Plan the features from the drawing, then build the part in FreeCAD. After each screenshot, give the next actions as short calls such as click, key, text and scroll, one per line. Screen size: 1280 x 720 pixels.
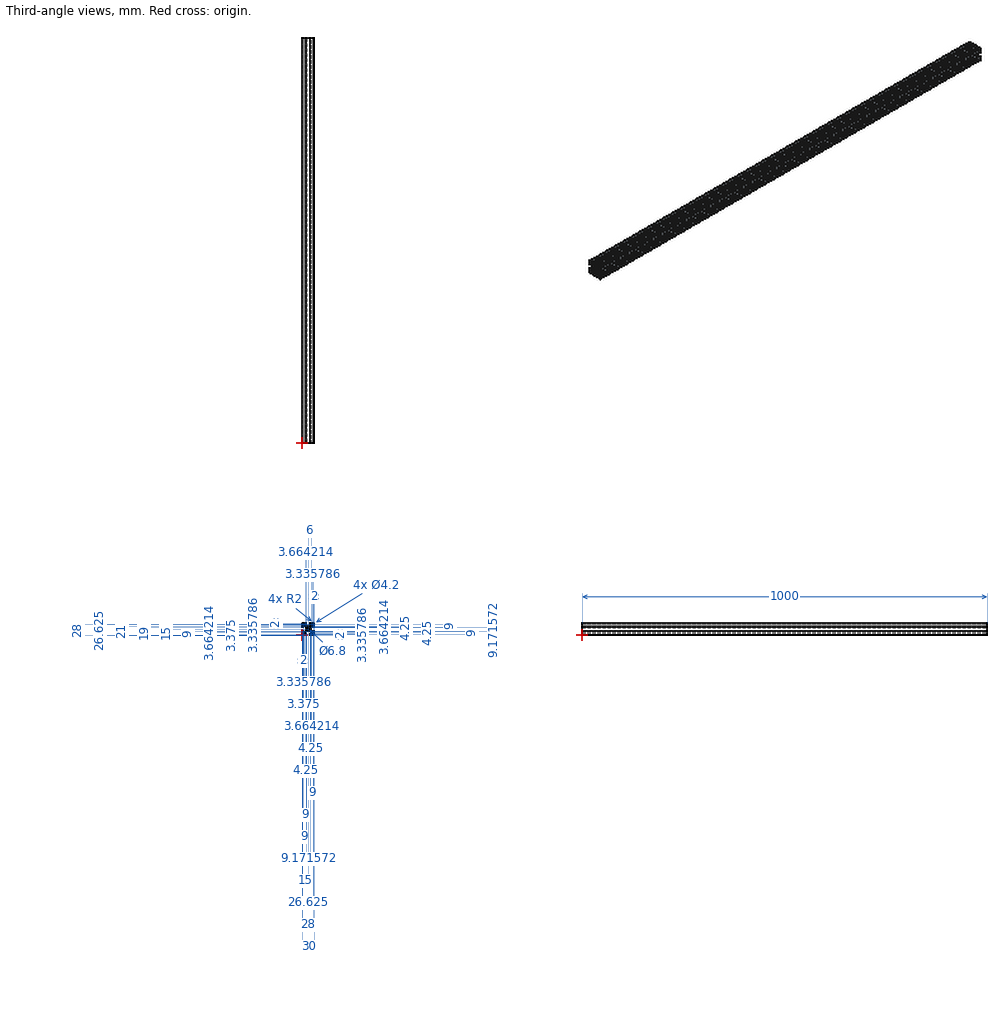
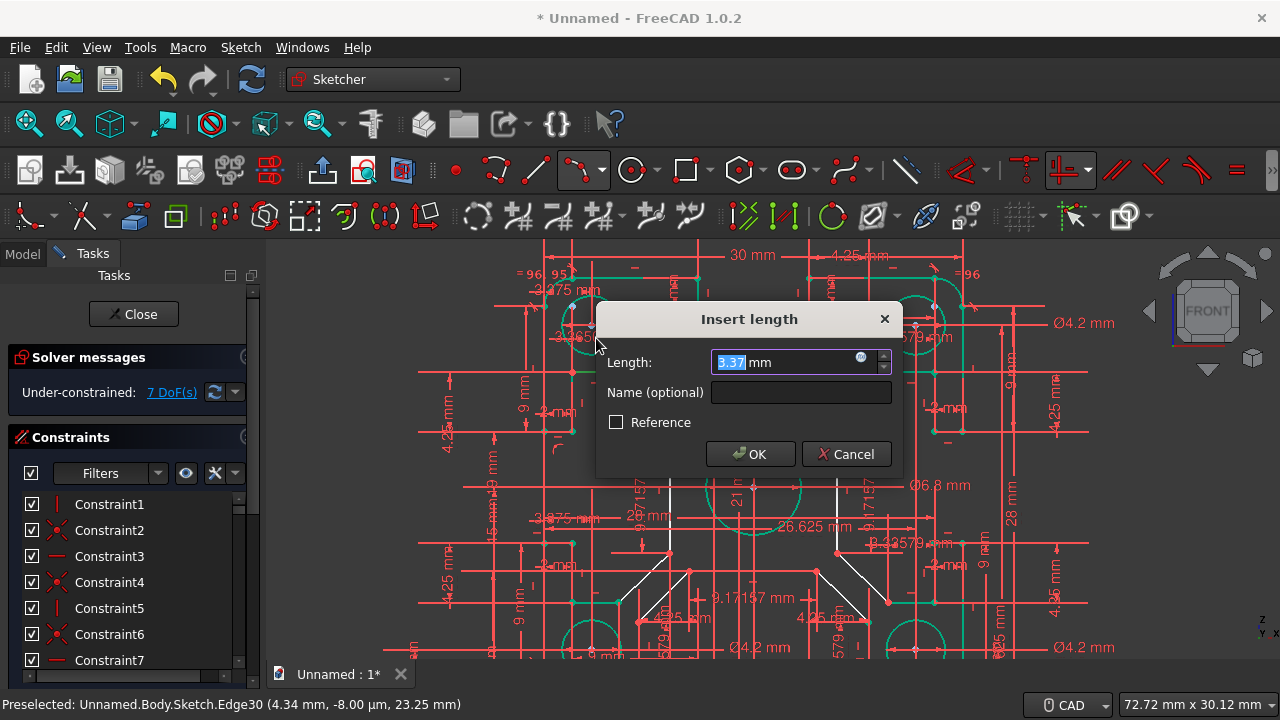
text(3.335786)
key(Return)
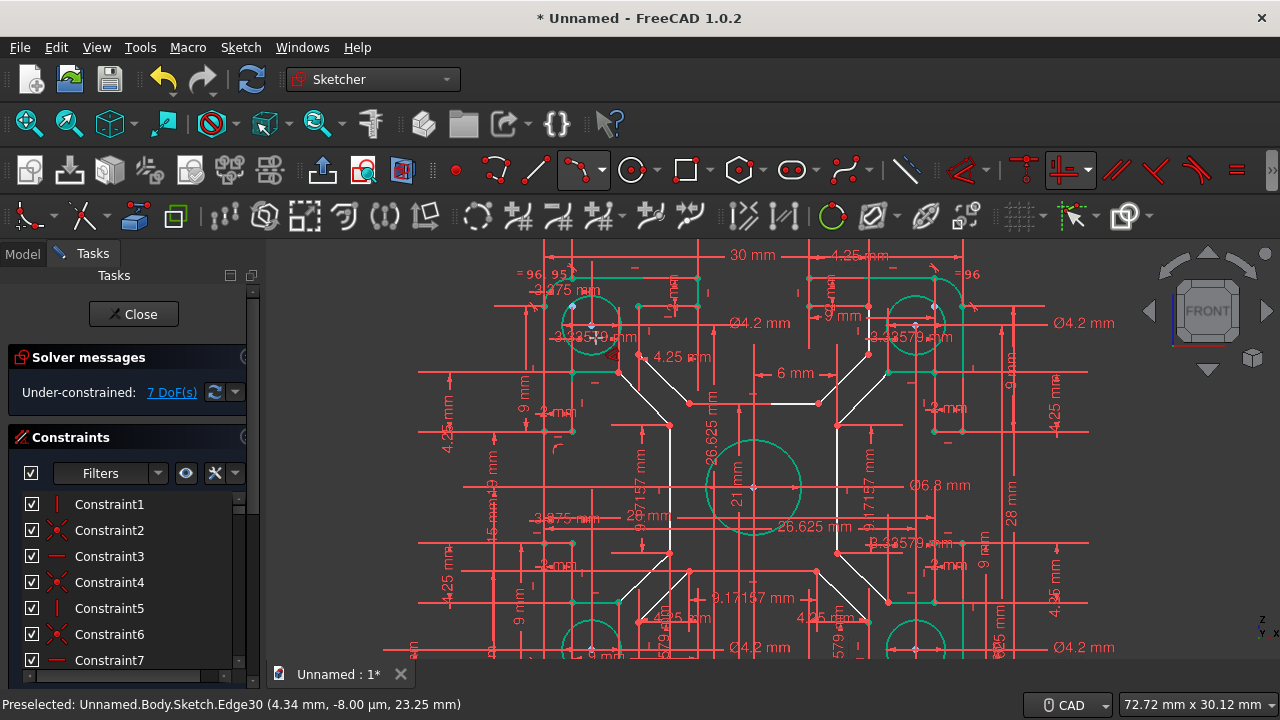
click(639, 321)
click(673, 330)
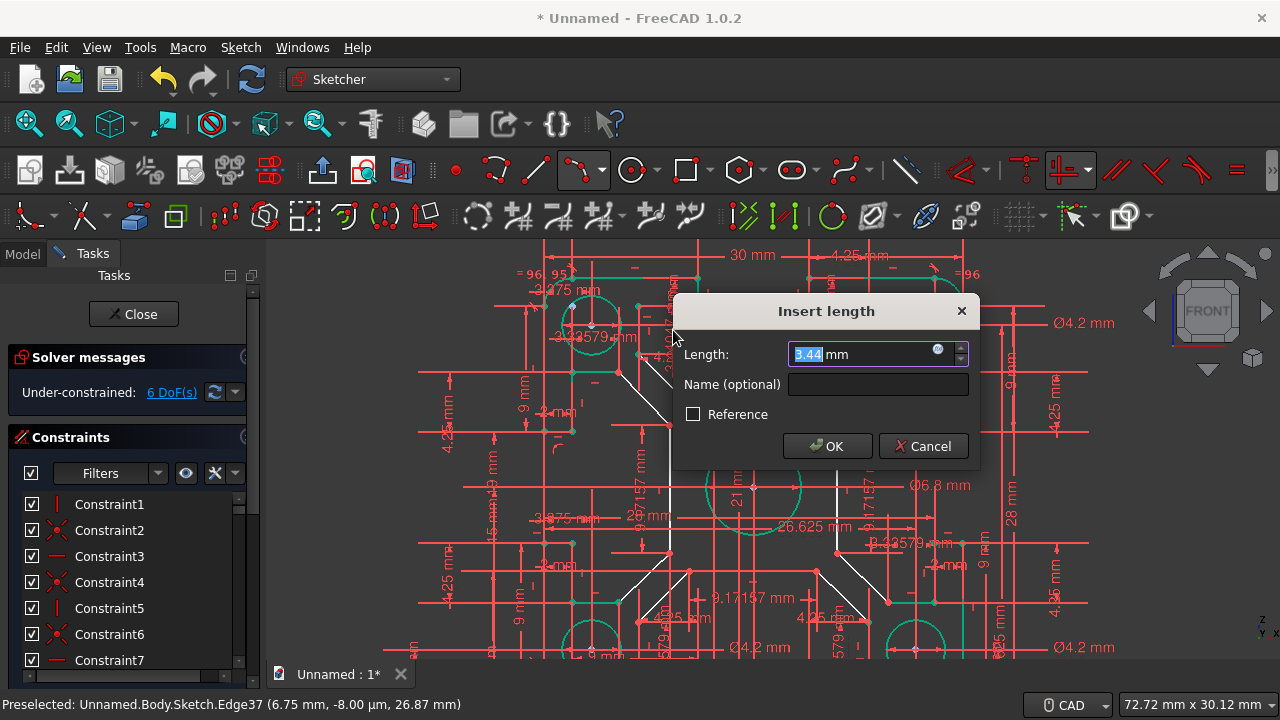
text(3.335786)
key(Return)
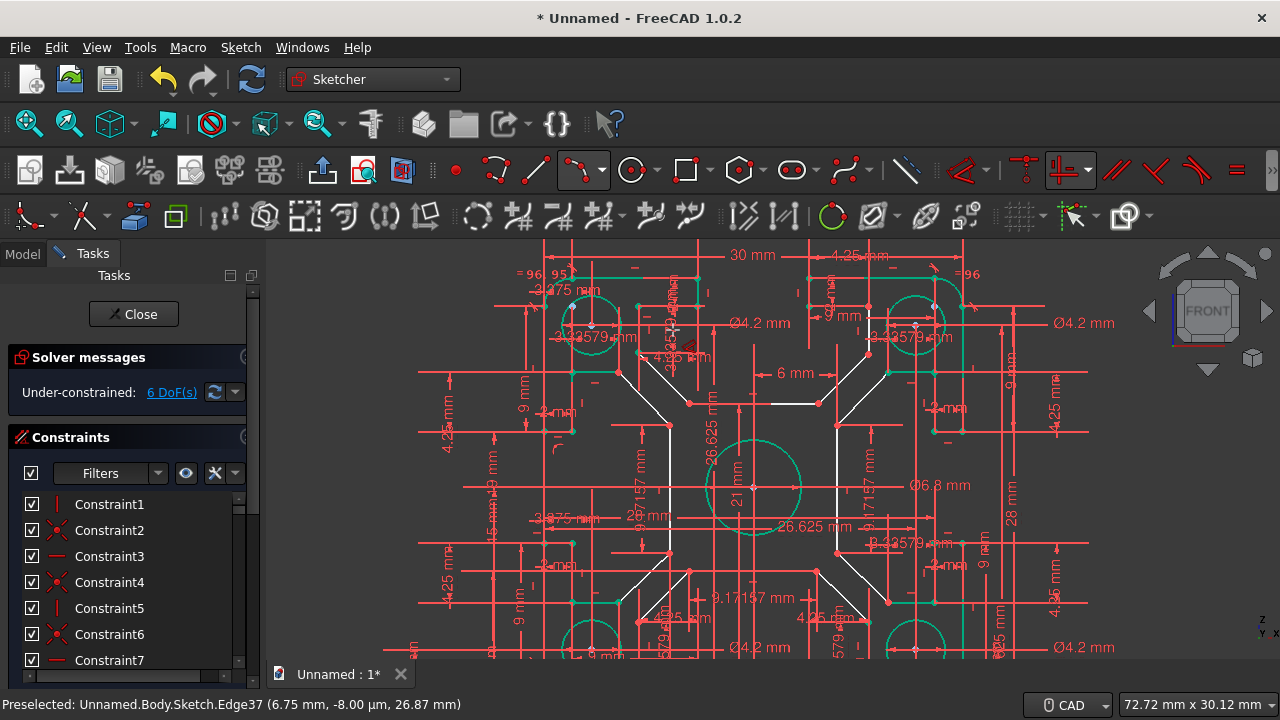
click(728, 404)
click(799, 438)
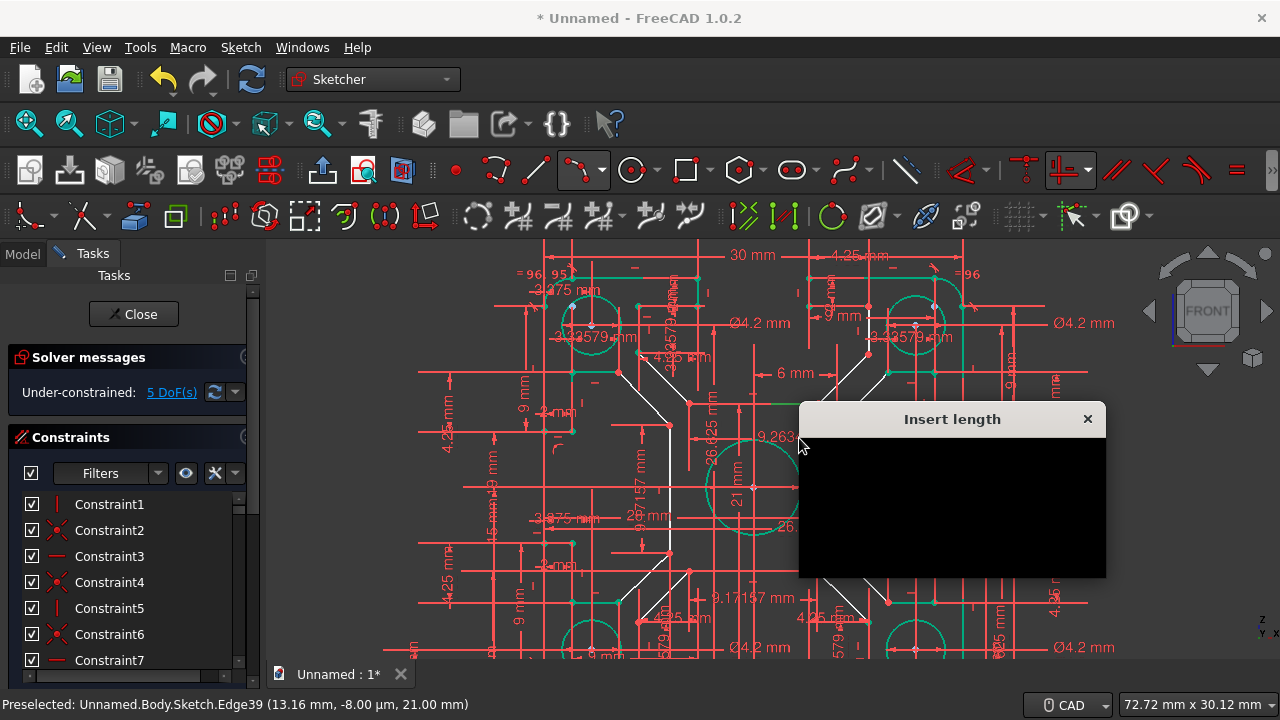
text(9.171572)
key(Return)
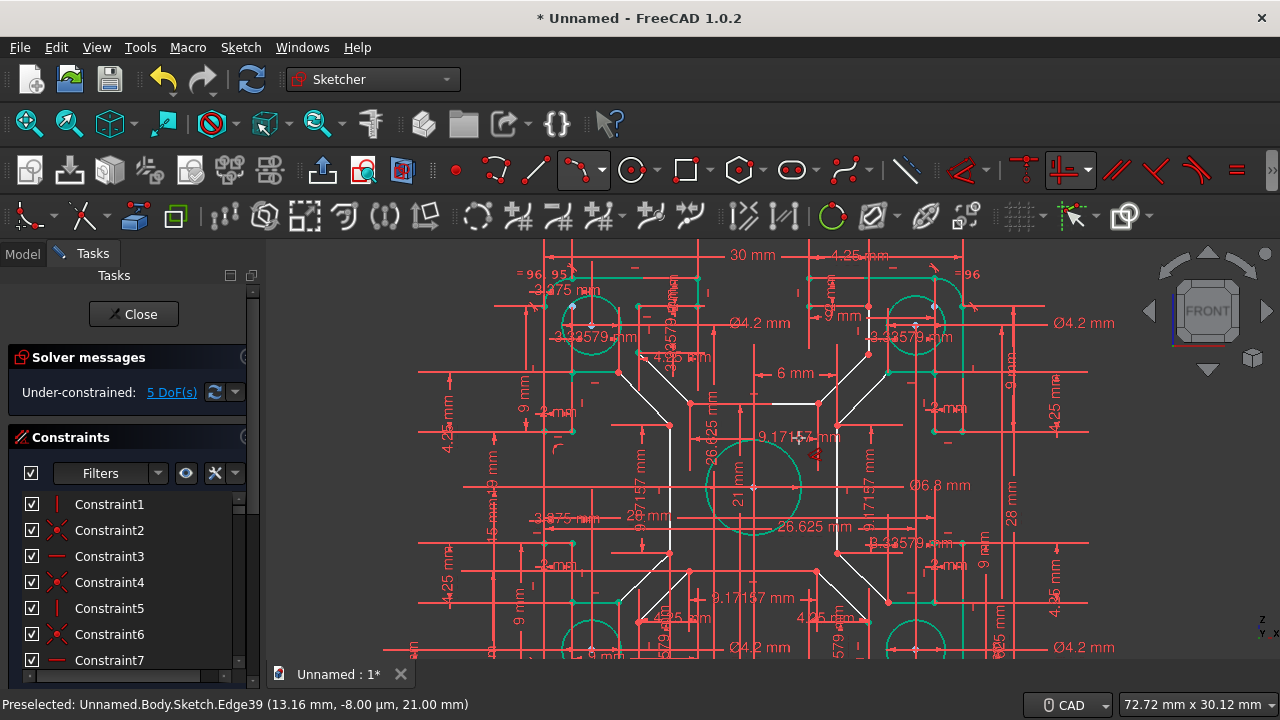
click(869, 340)
click(835, 341)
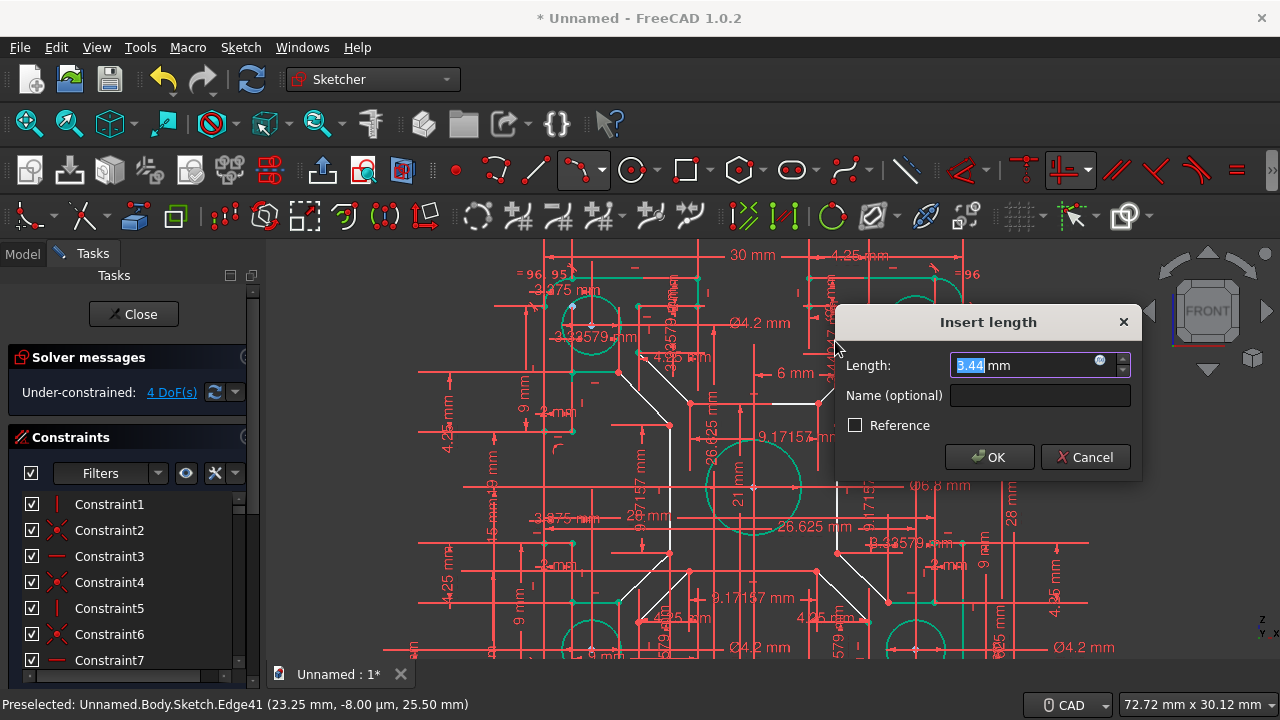
text(3.335786)
key(Return)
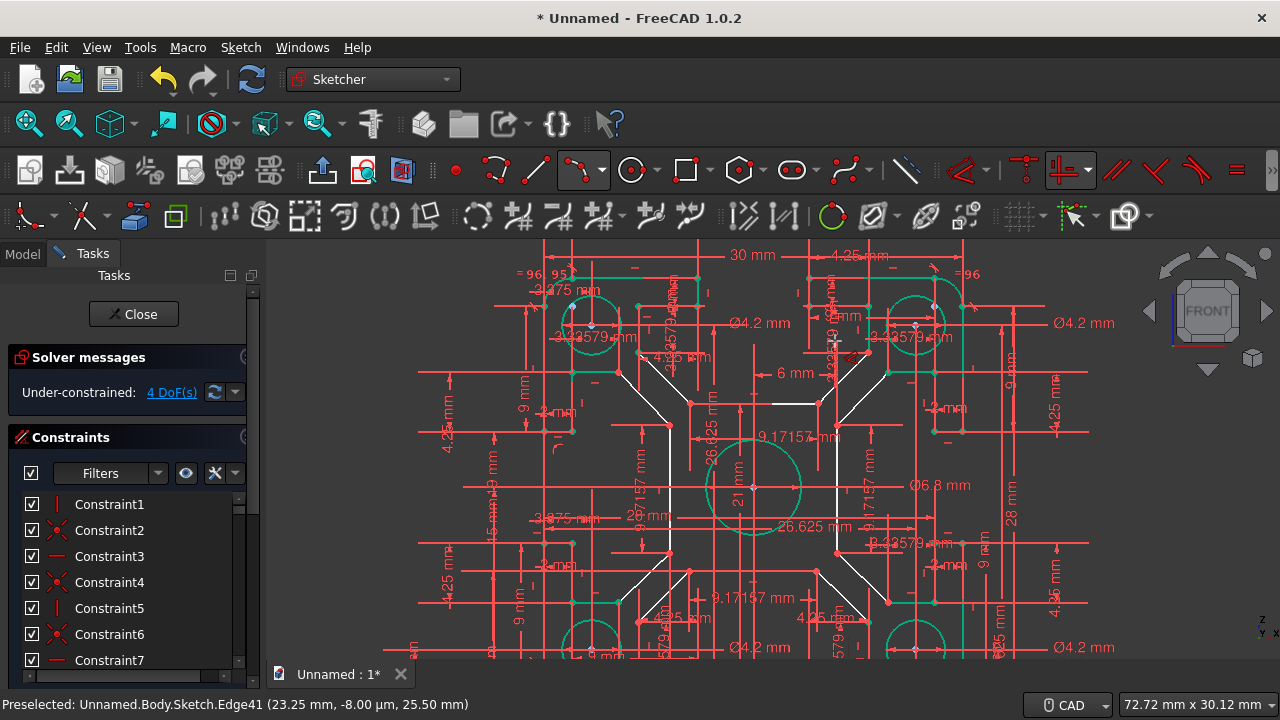
click(873, 388)
click(803, 417)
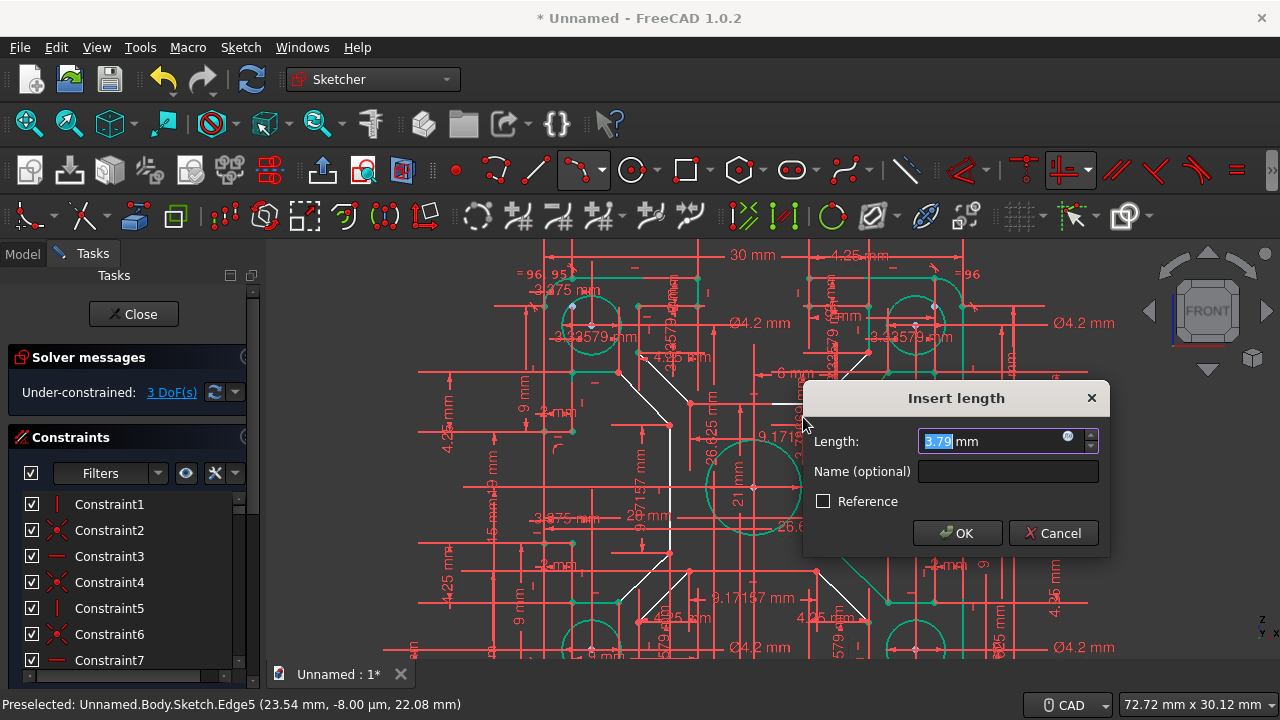
text(3.664214)
key(Return)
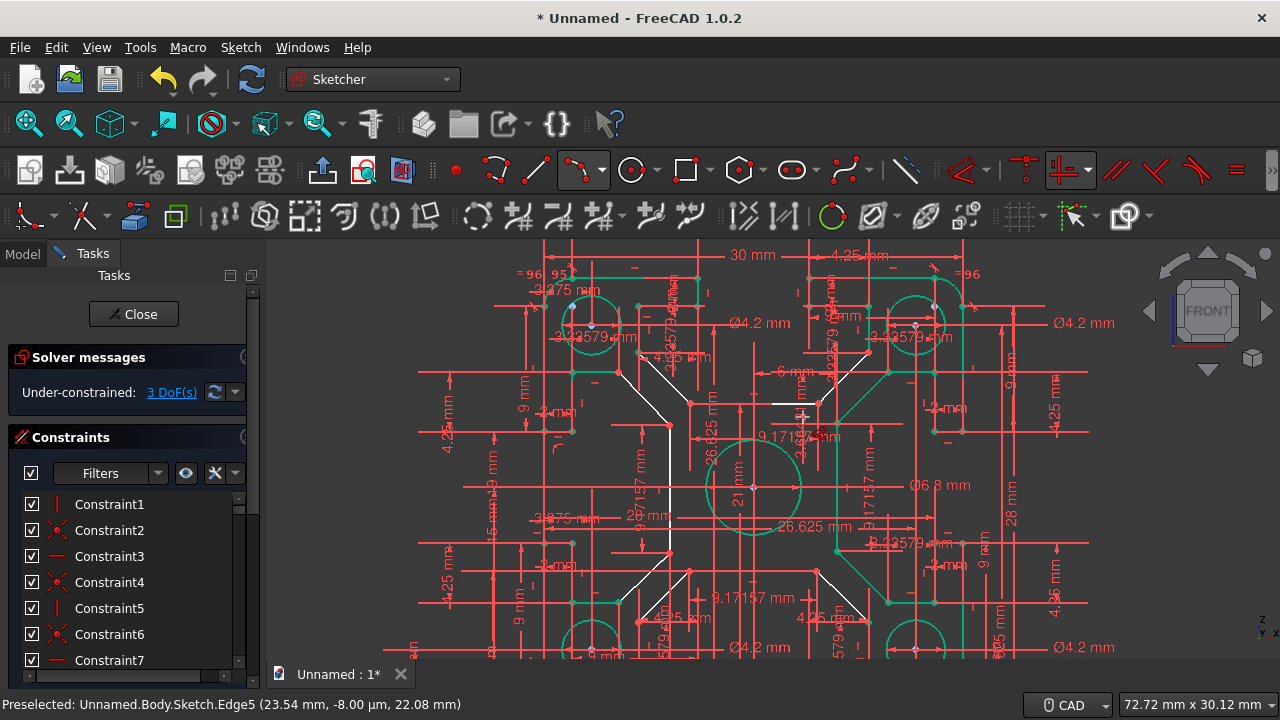
click(853, 607)
click(855, 465)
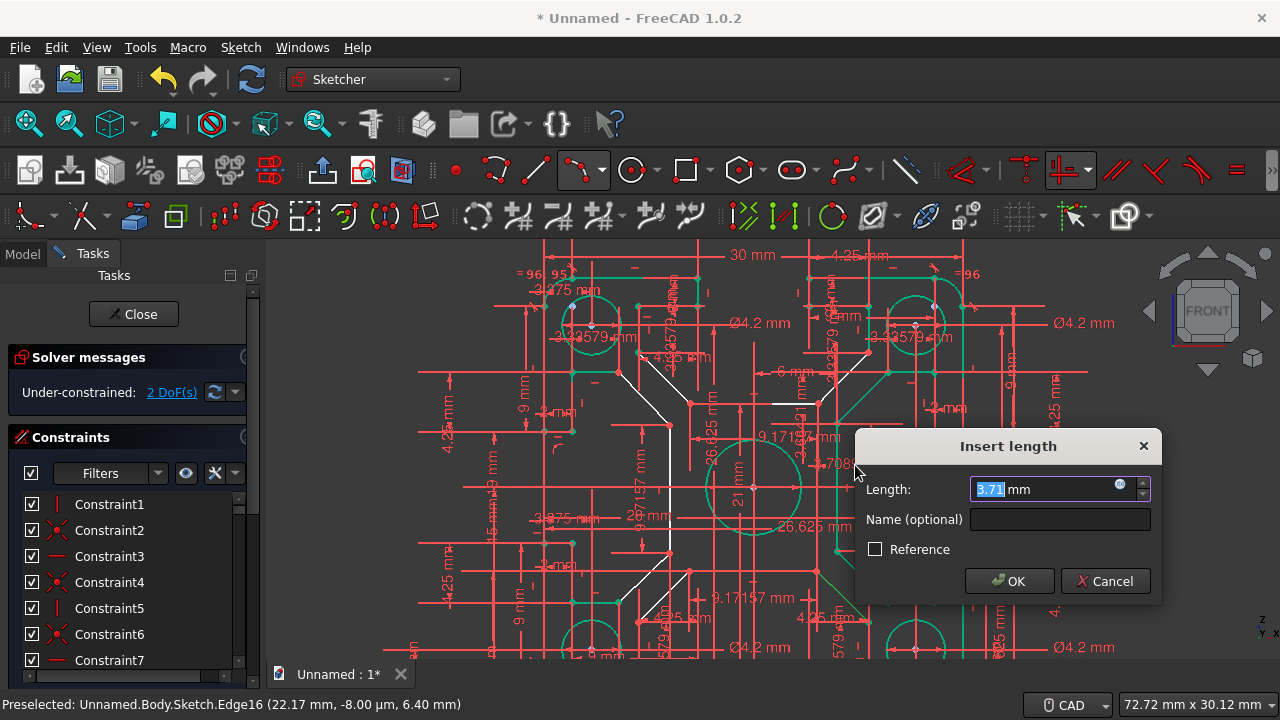
text(3.664214)
key(Return)